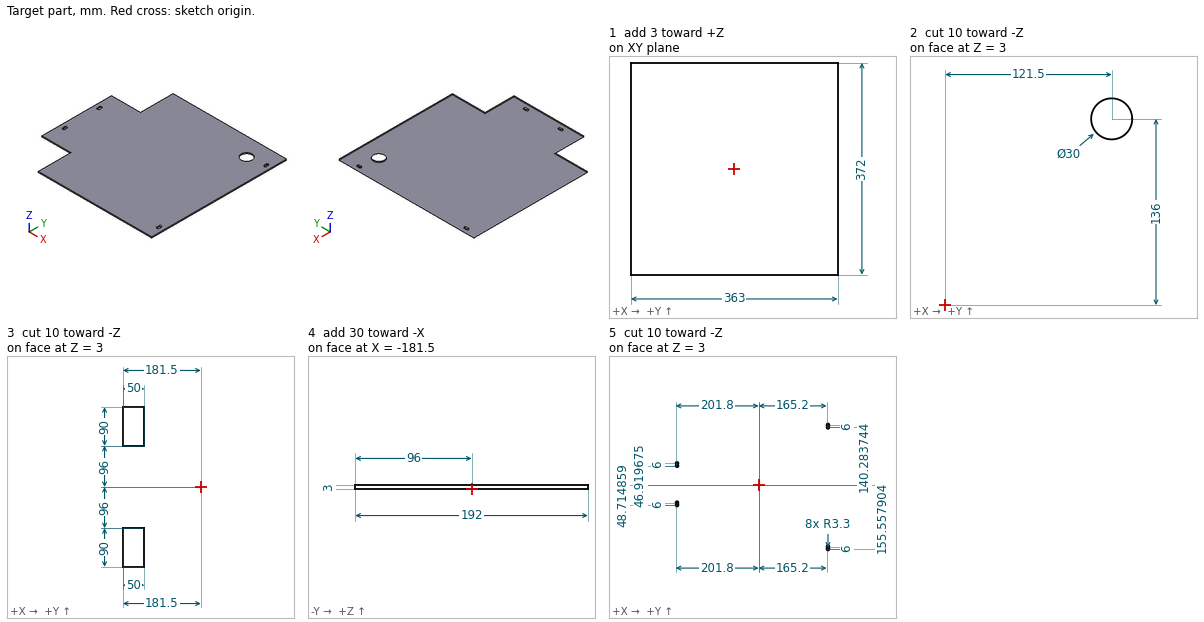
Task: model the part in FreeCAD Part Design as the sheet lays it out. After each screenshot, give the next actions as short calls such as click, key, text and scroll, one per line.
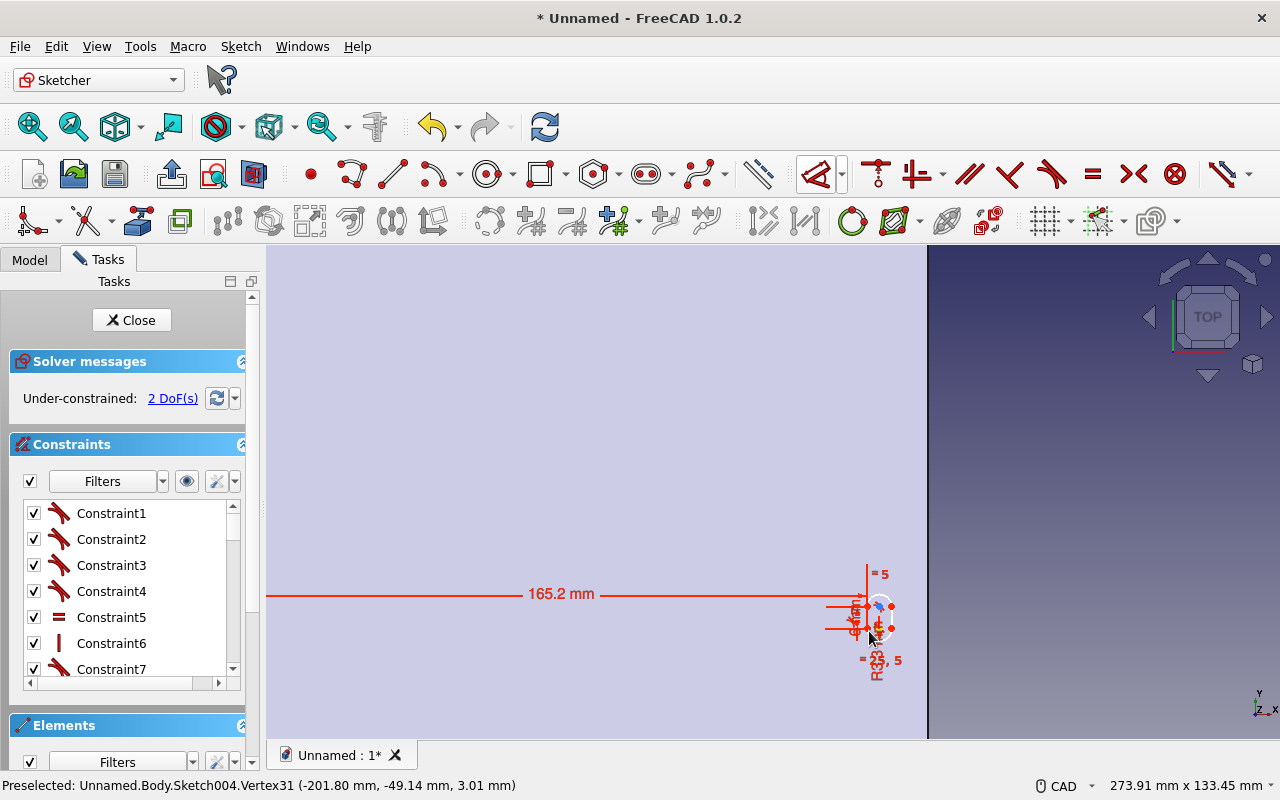
click(867, 629)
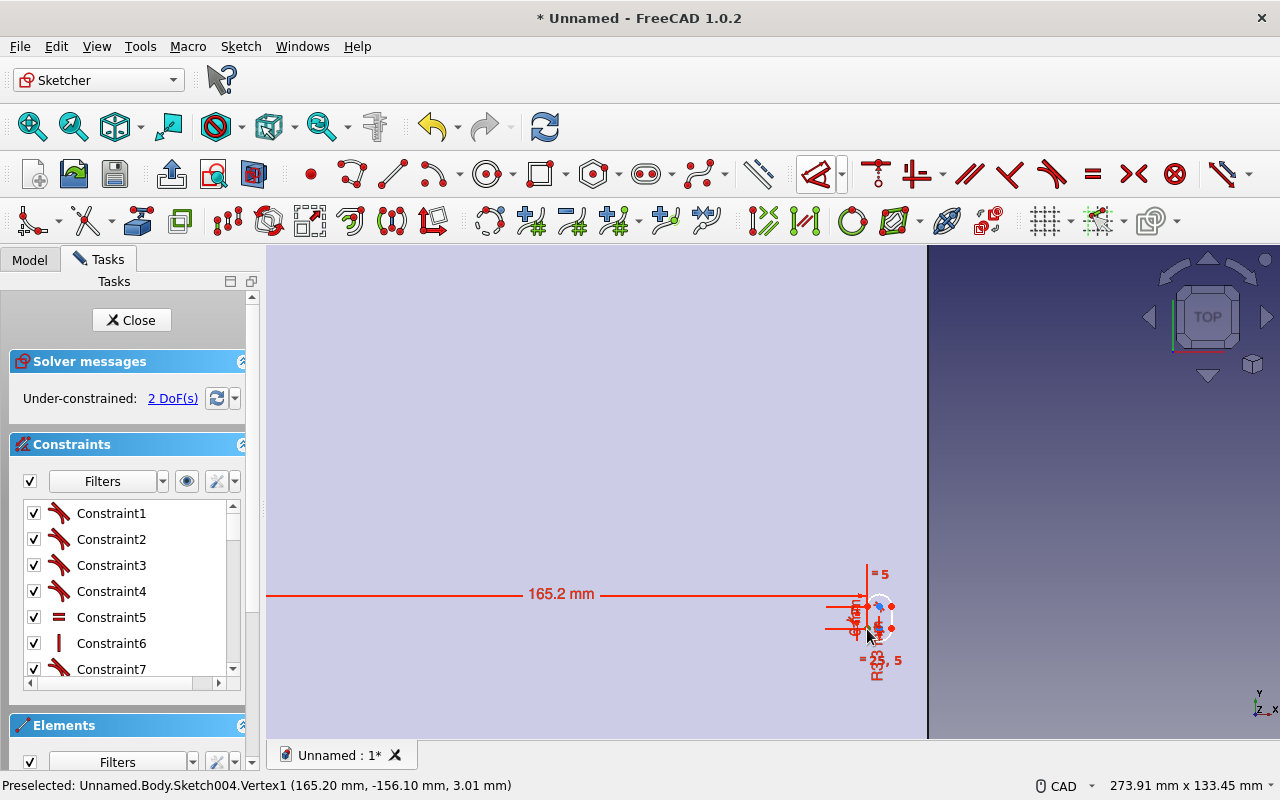
key(i)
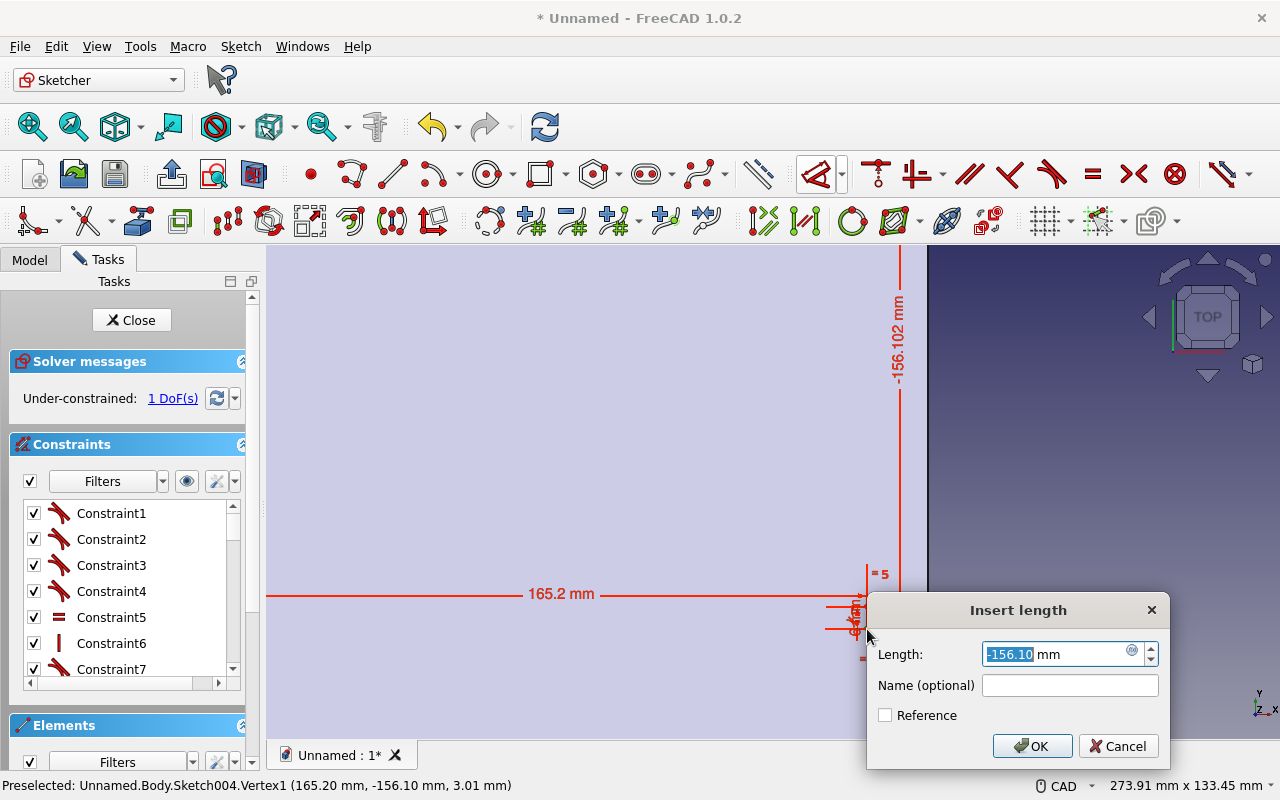
text(-155.557904)
key(Return)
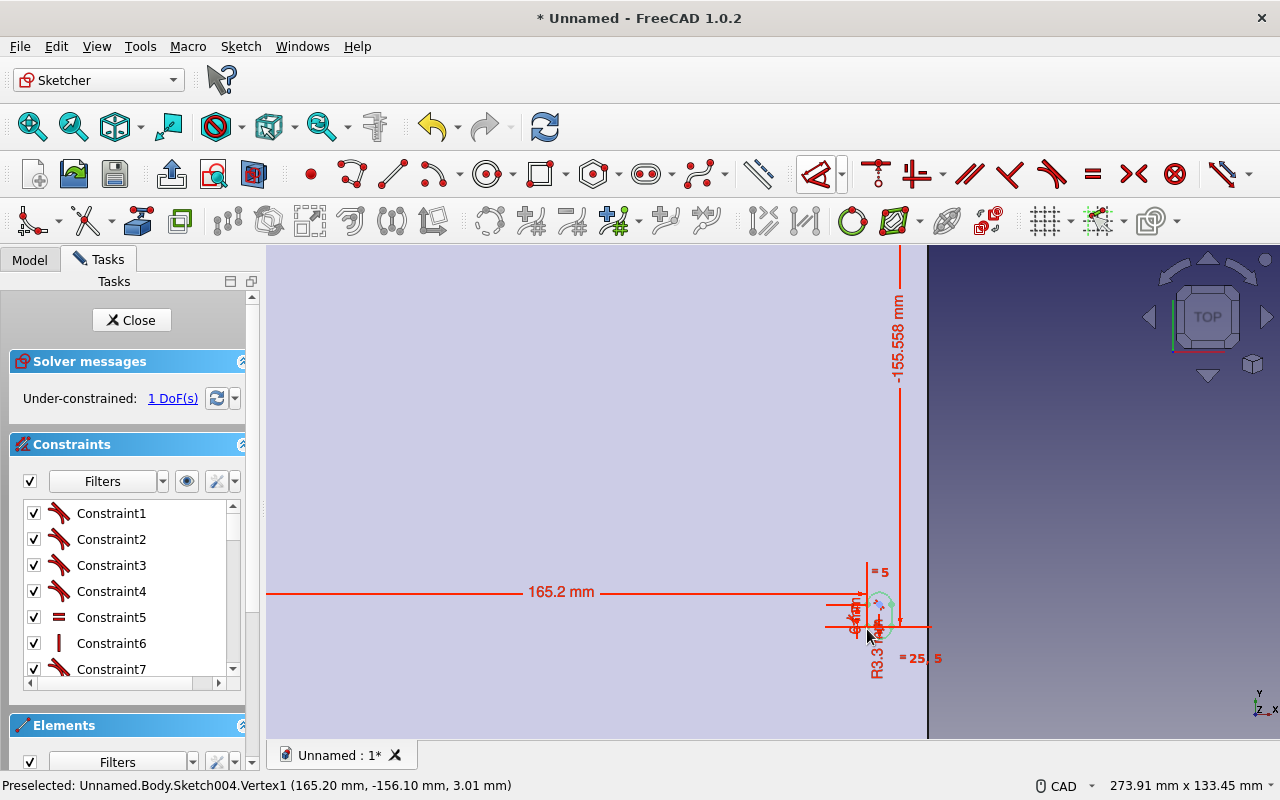
scroll(870, 631, down, 7)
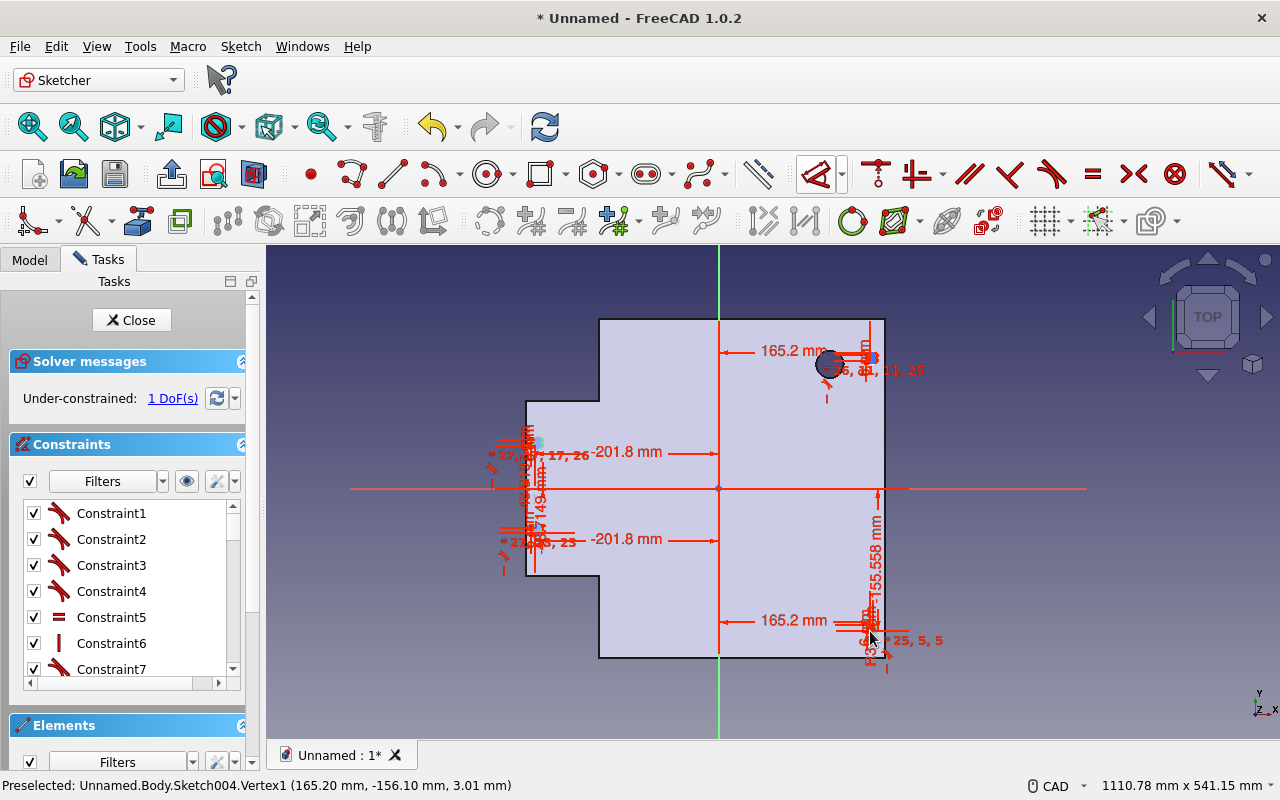
scroll(870, 361, up, 7)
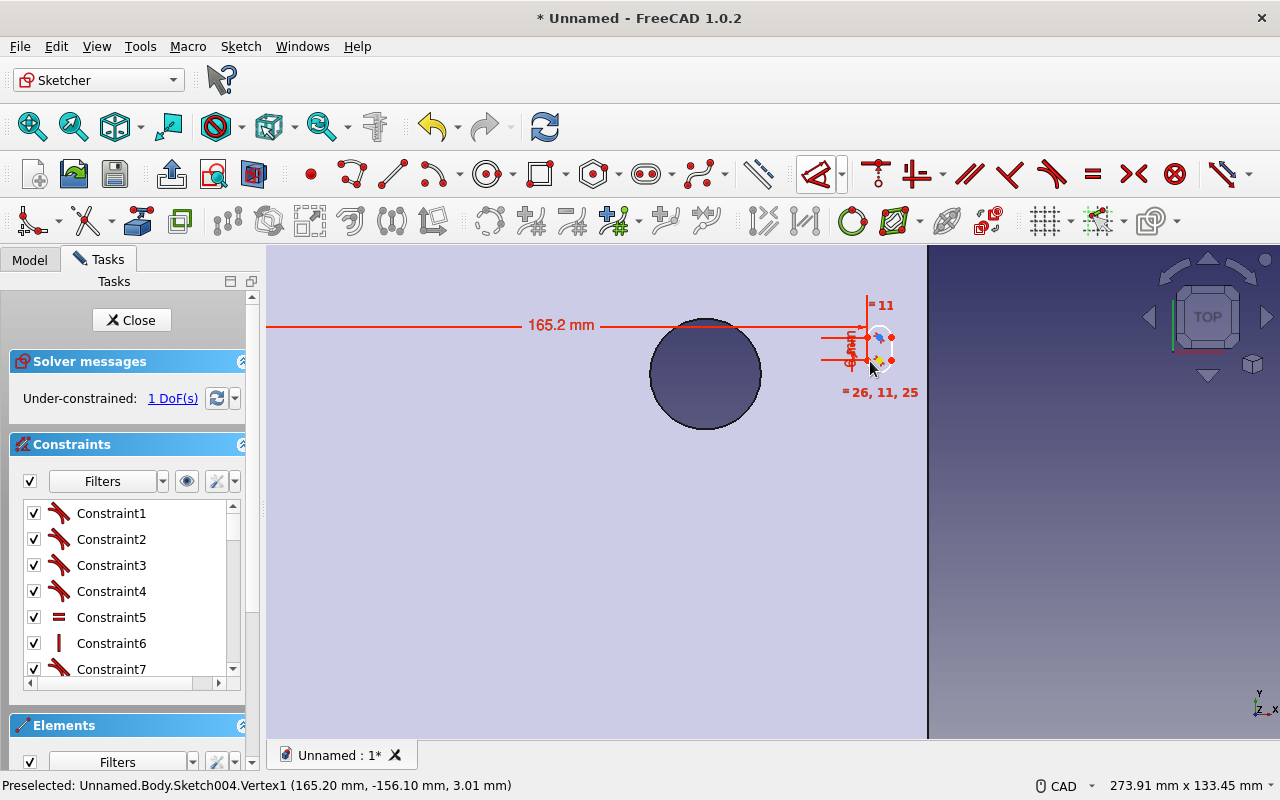
click(867, 360)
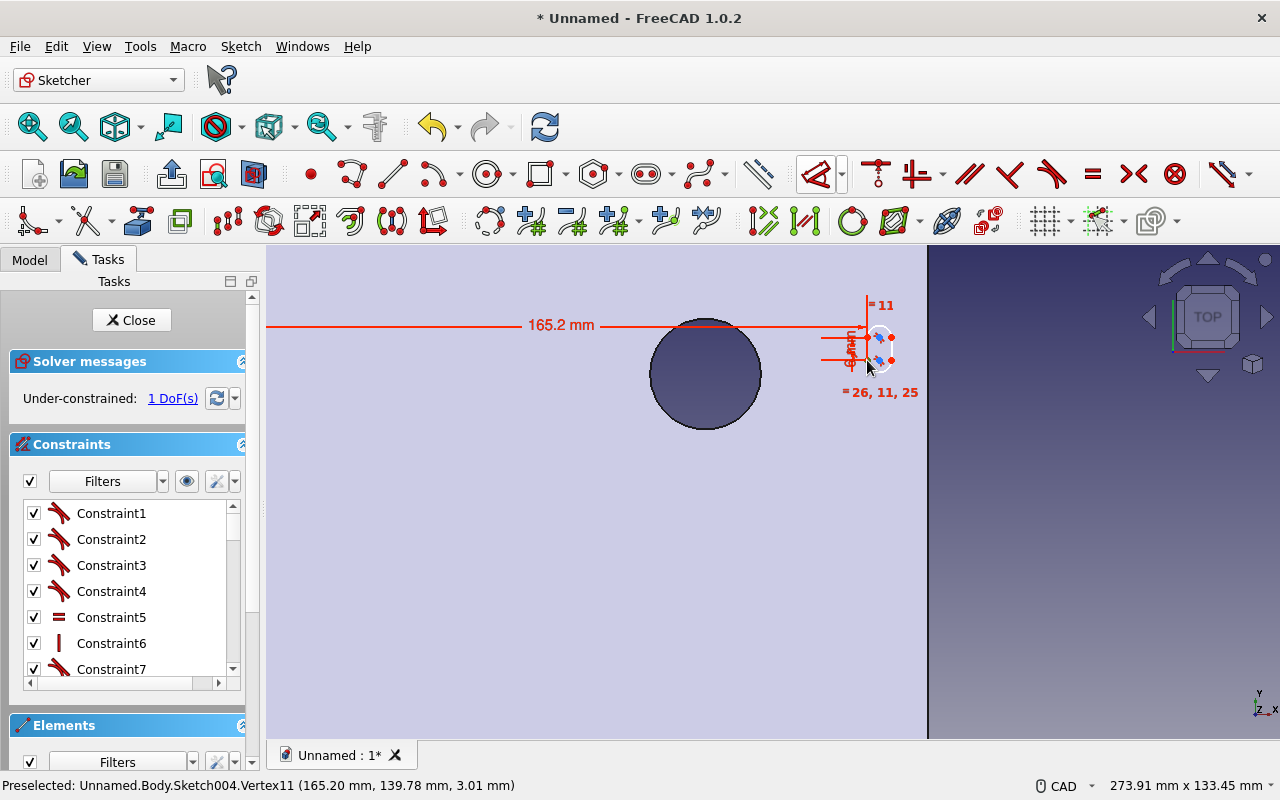
key(i)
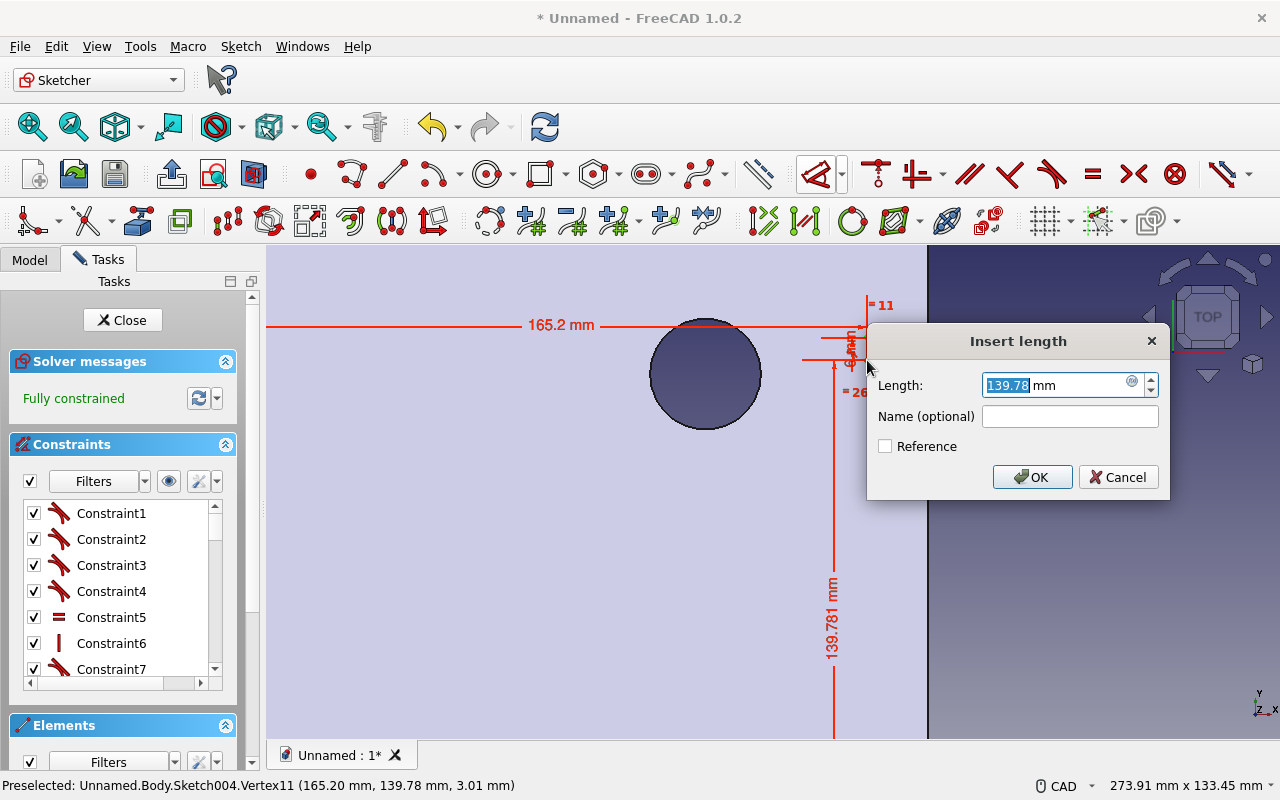
text(140.283744)
key(Return)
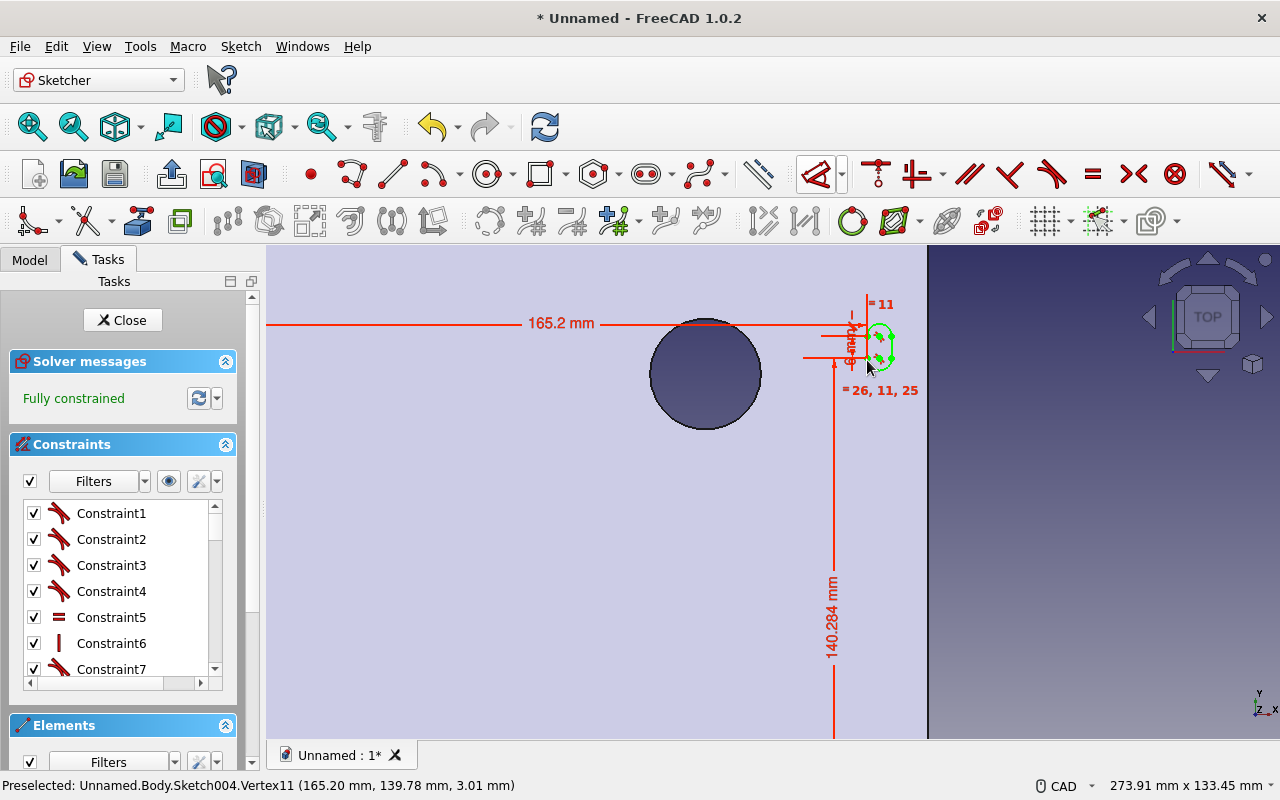
click(123, 320)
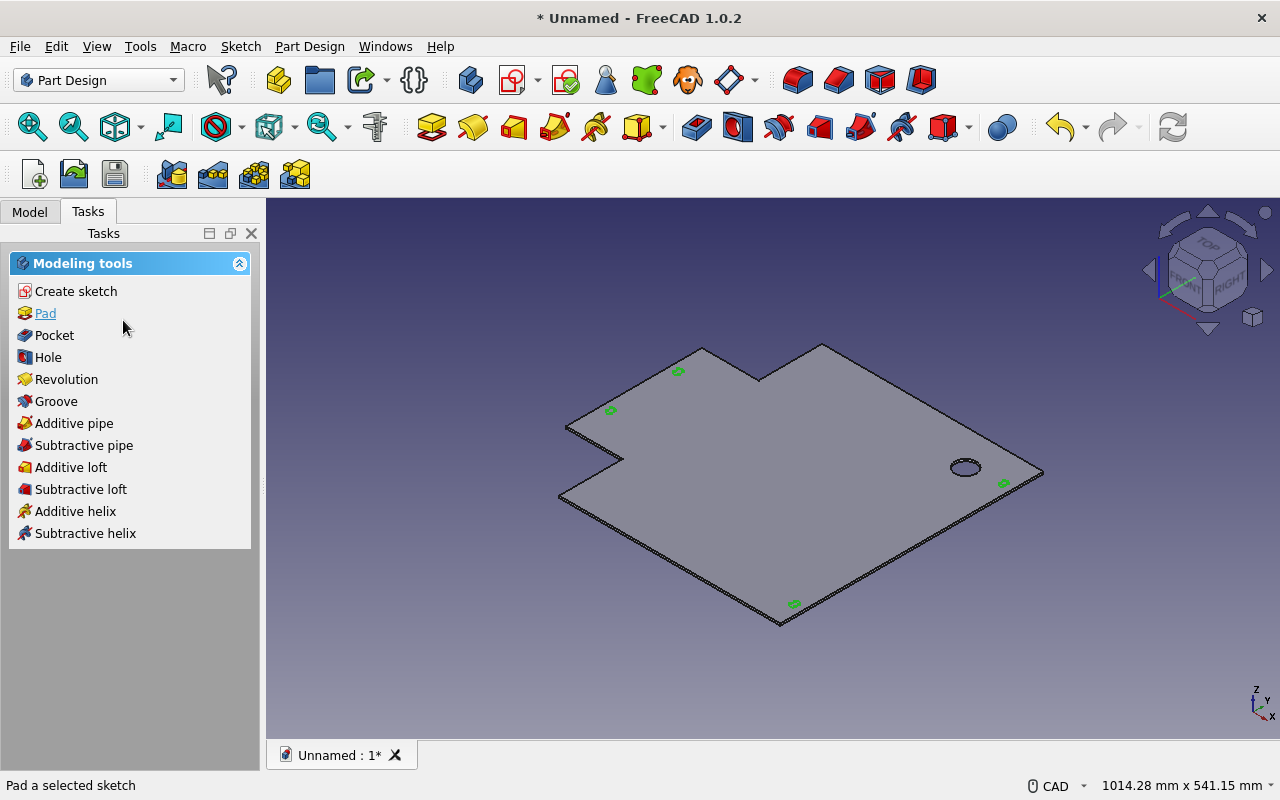
click(697, 128)